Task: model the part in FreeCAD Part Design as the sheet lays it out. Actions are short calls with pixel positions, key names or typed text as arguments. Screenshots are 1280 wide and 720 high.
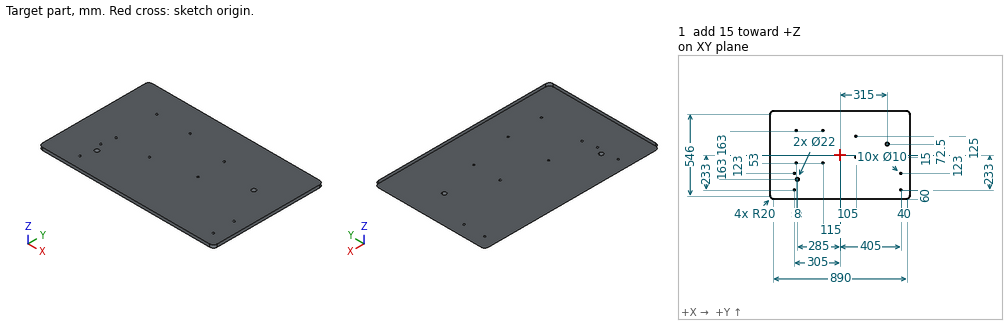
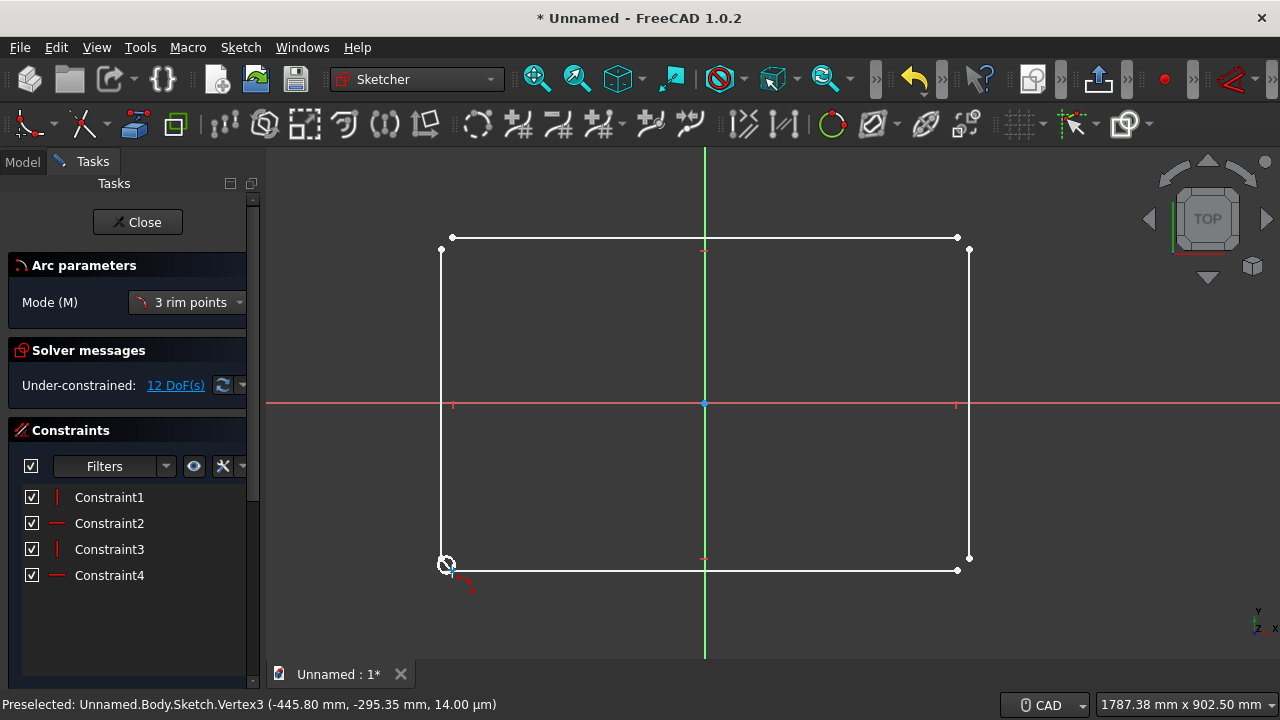
scroll(444, 566, up, 8)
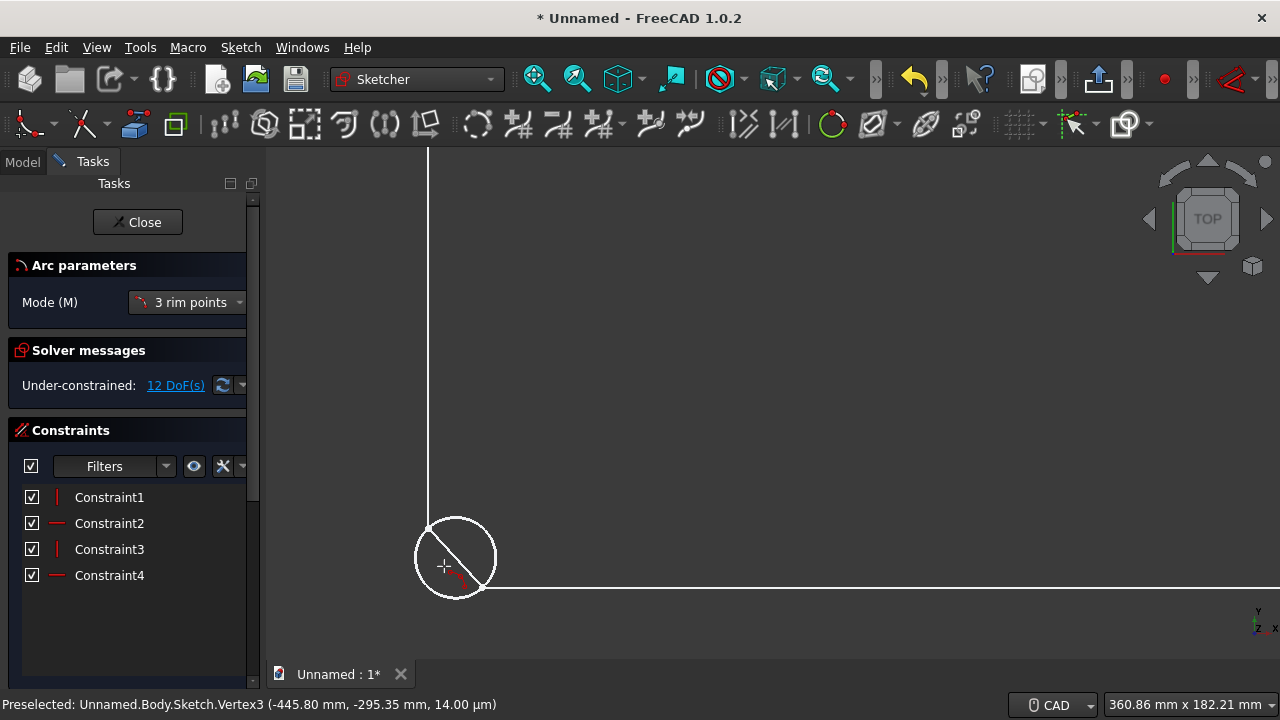
click(445, 564)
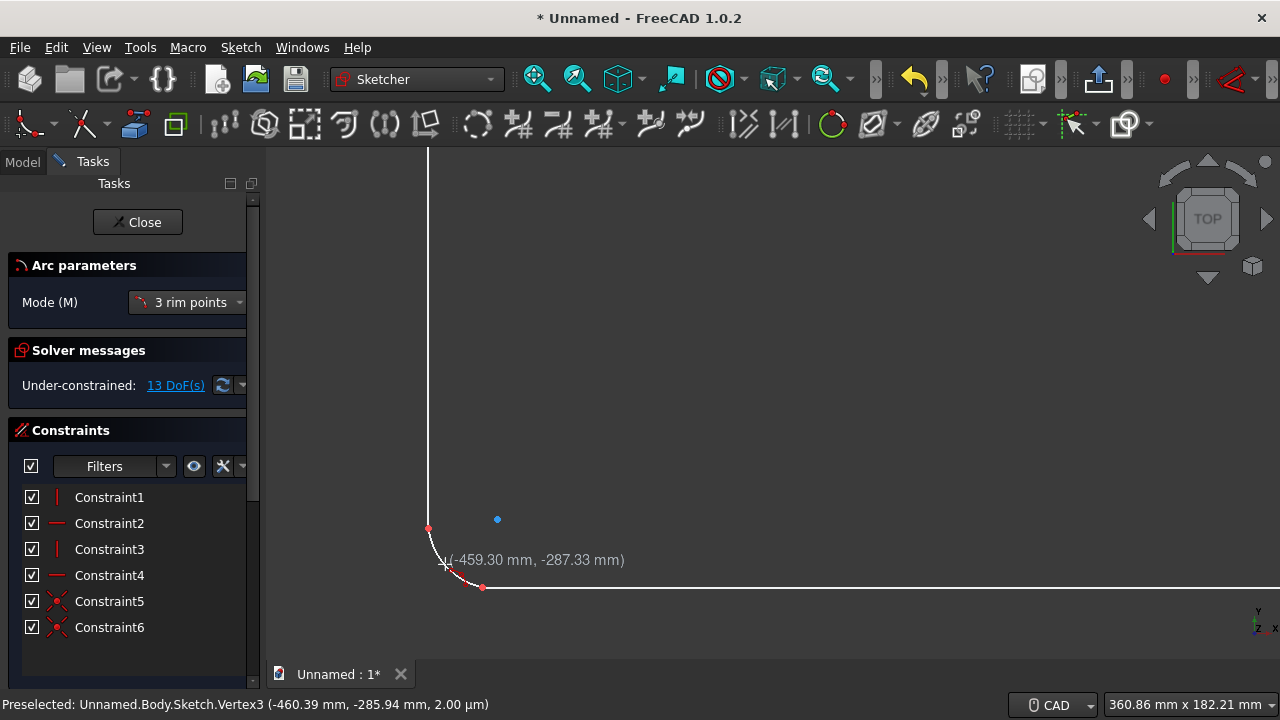
scroll(444, 566, down, 8)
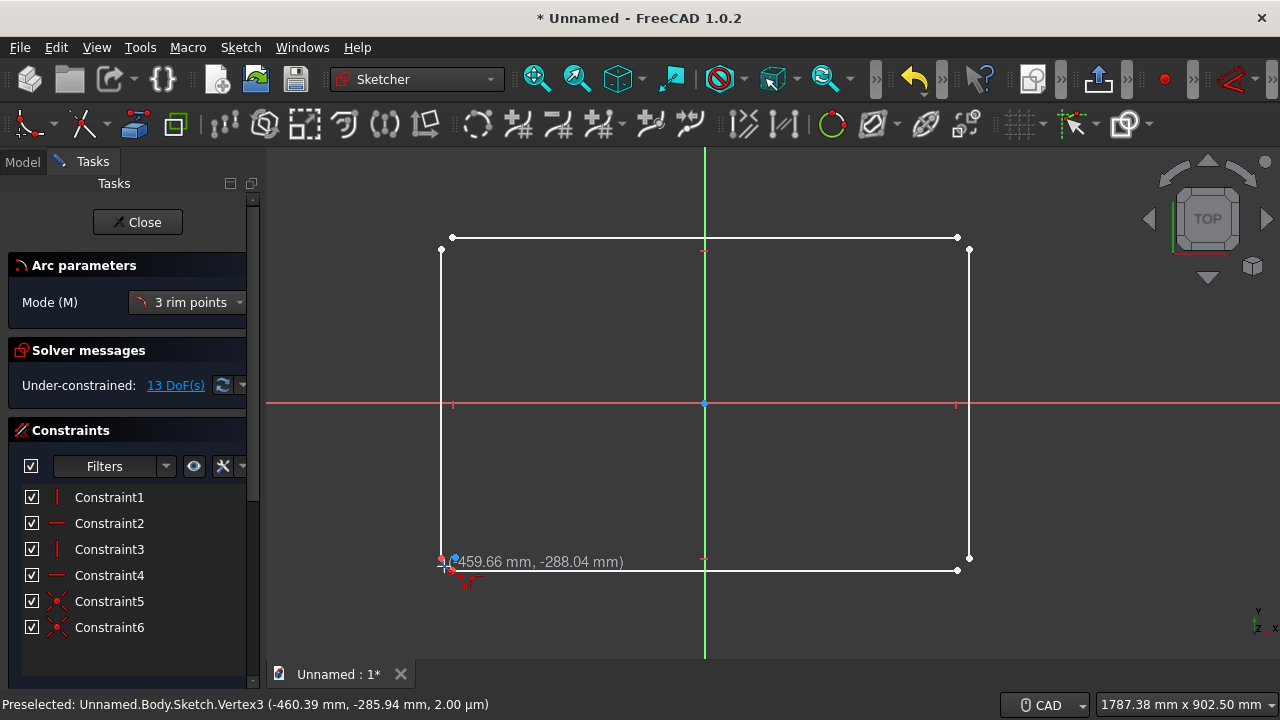
click(957, 571)
click(969, 559)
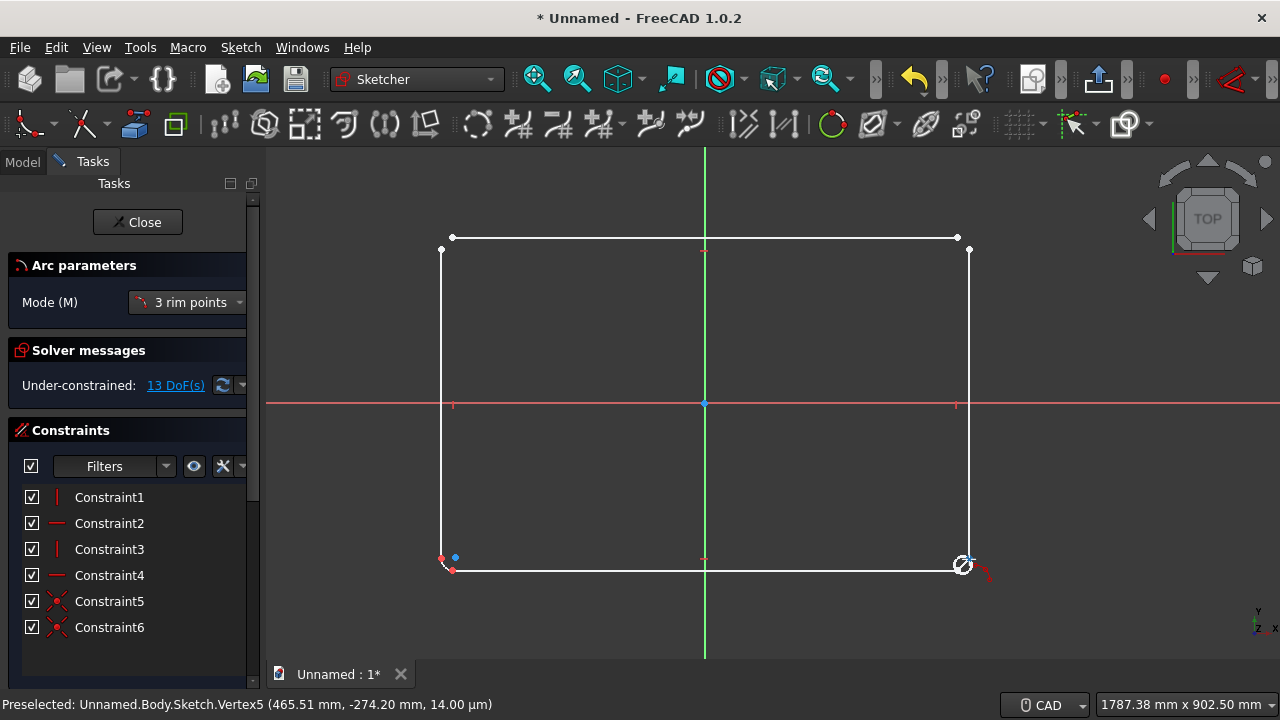
scroll(965, 566, up, 8)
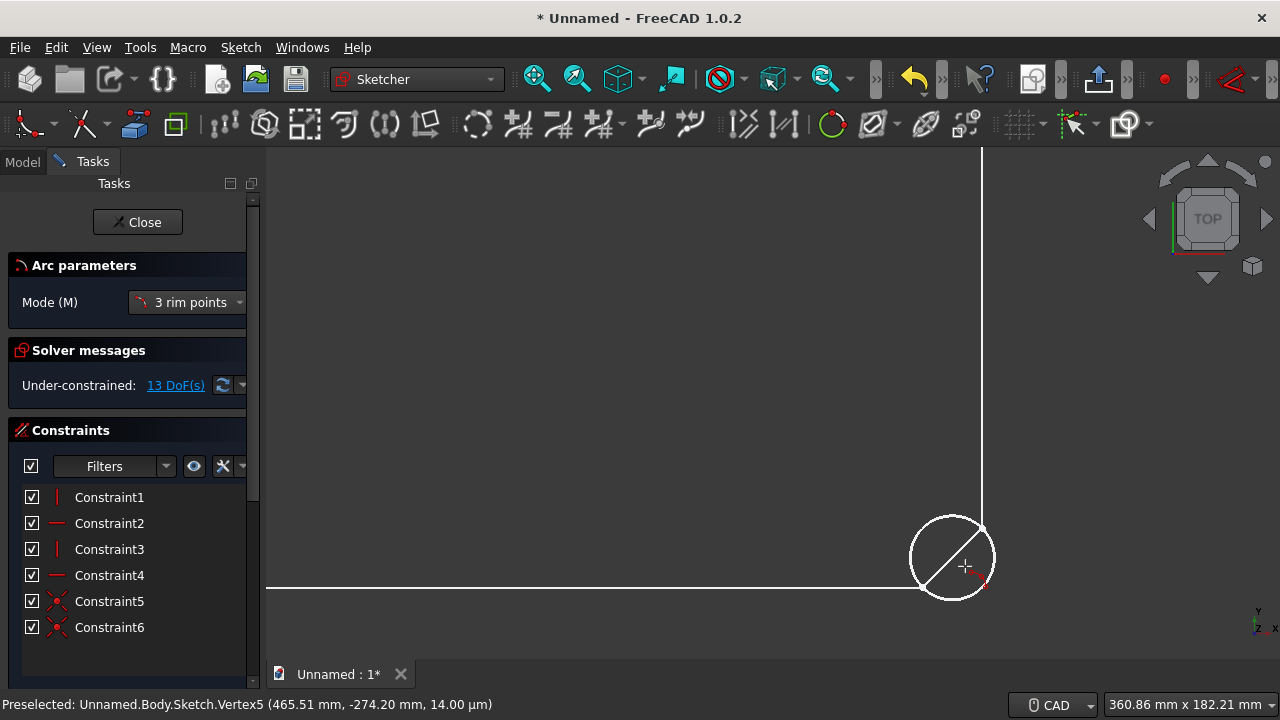
click(964, 564)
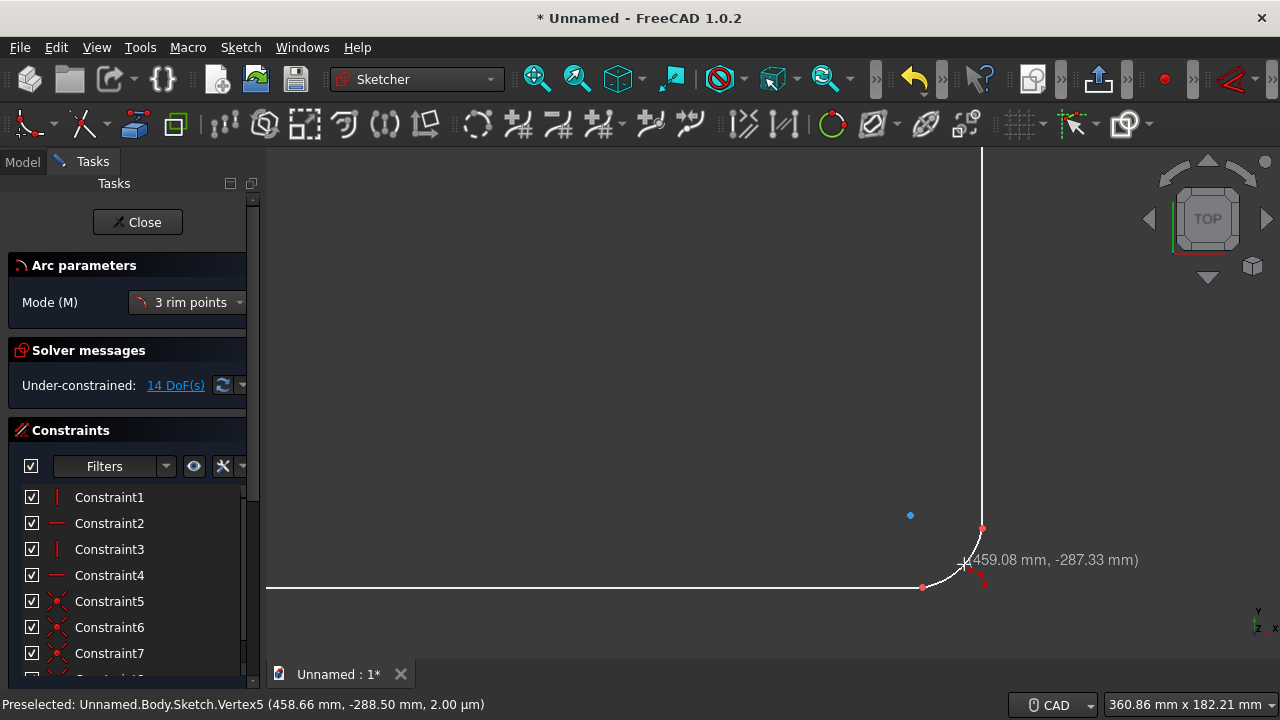
scroll(965, 566, down, 8)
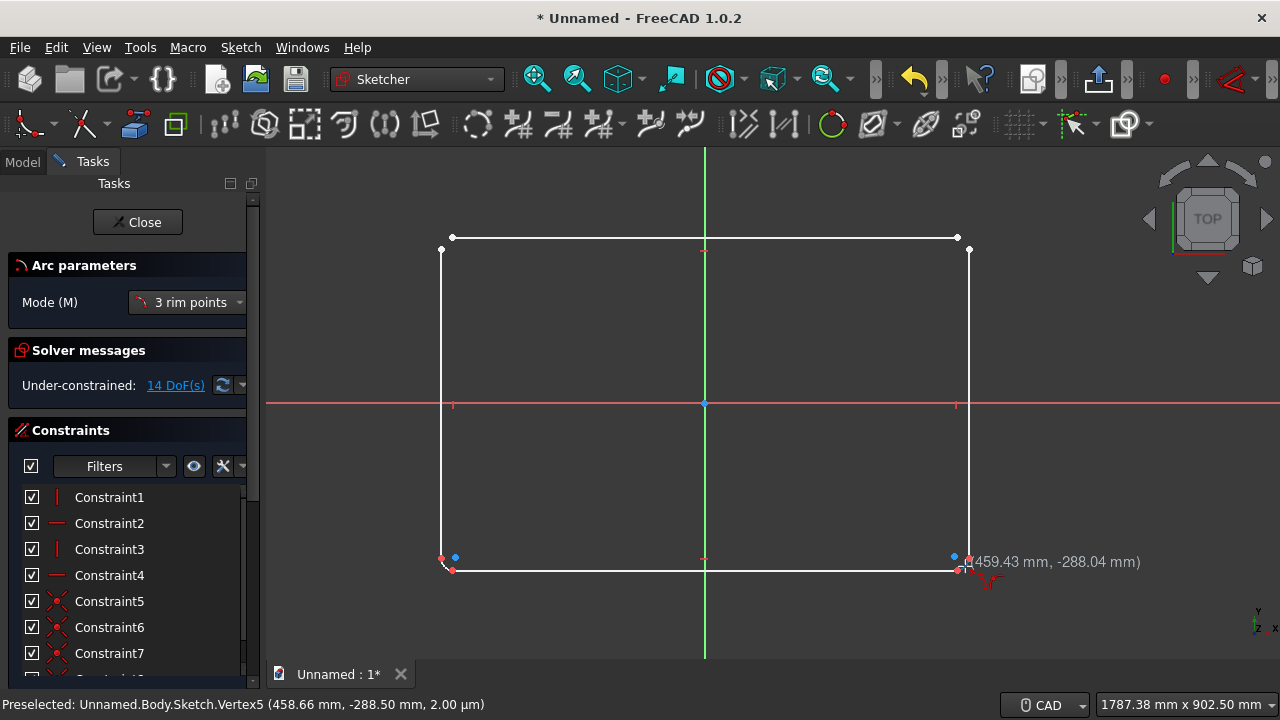
click(969, 250)
click(957, 238)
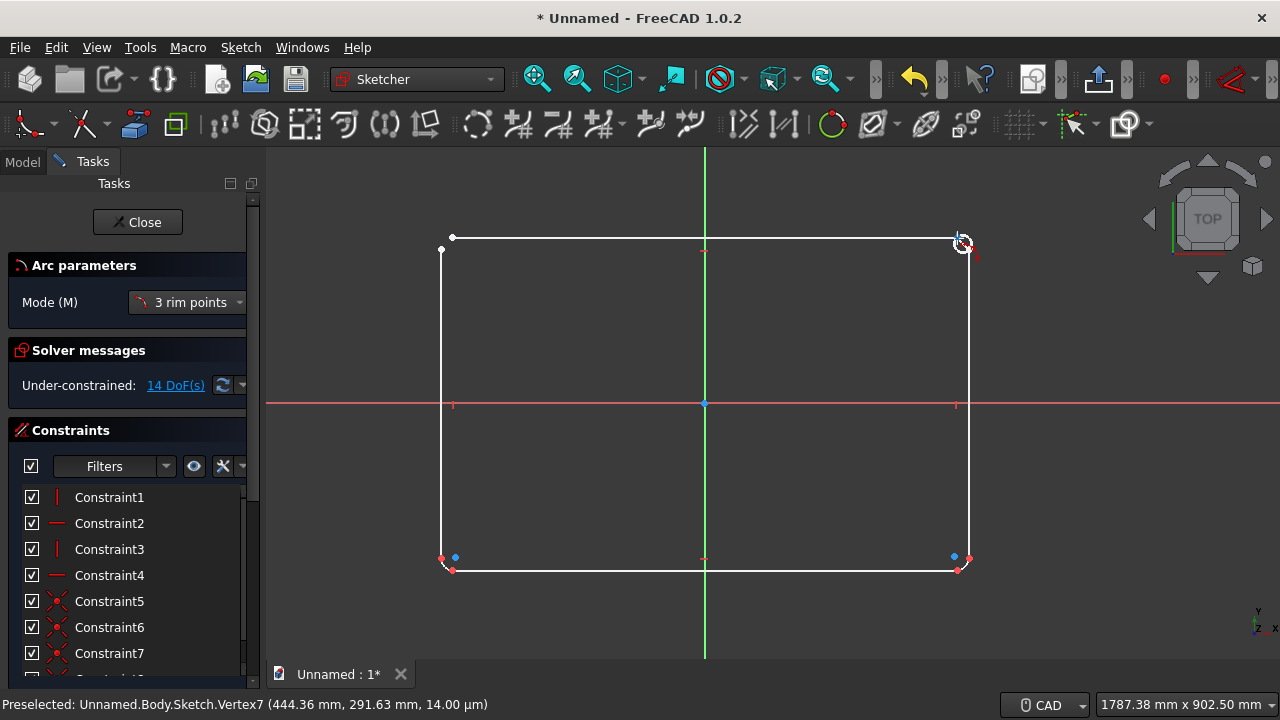
scroll(965, 241, up, 8)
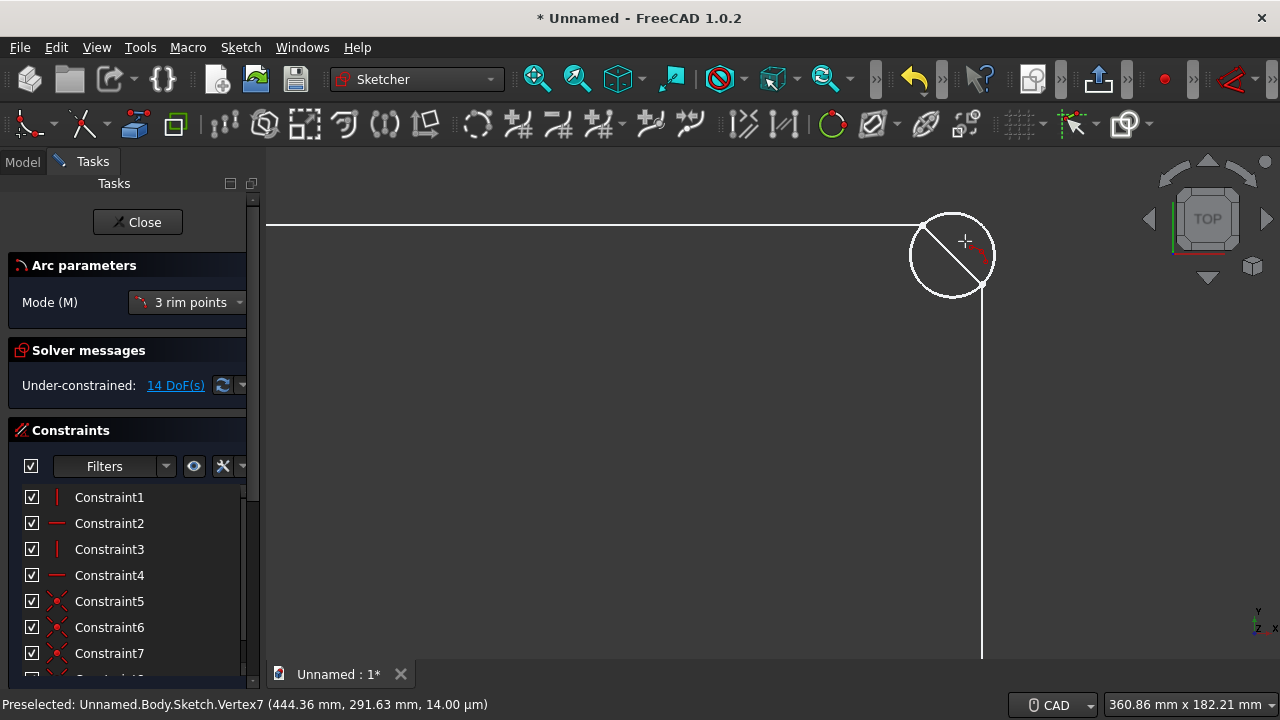
click(964, 238)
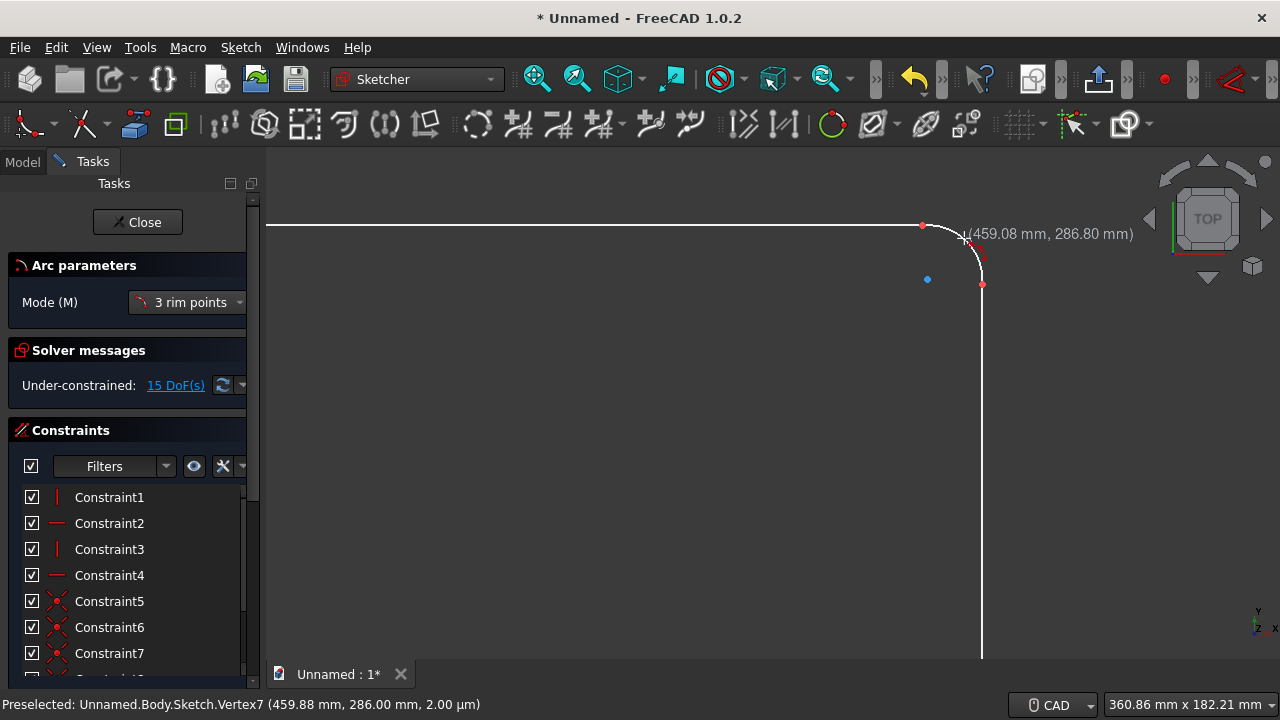
scroll(965, 241, down, 8)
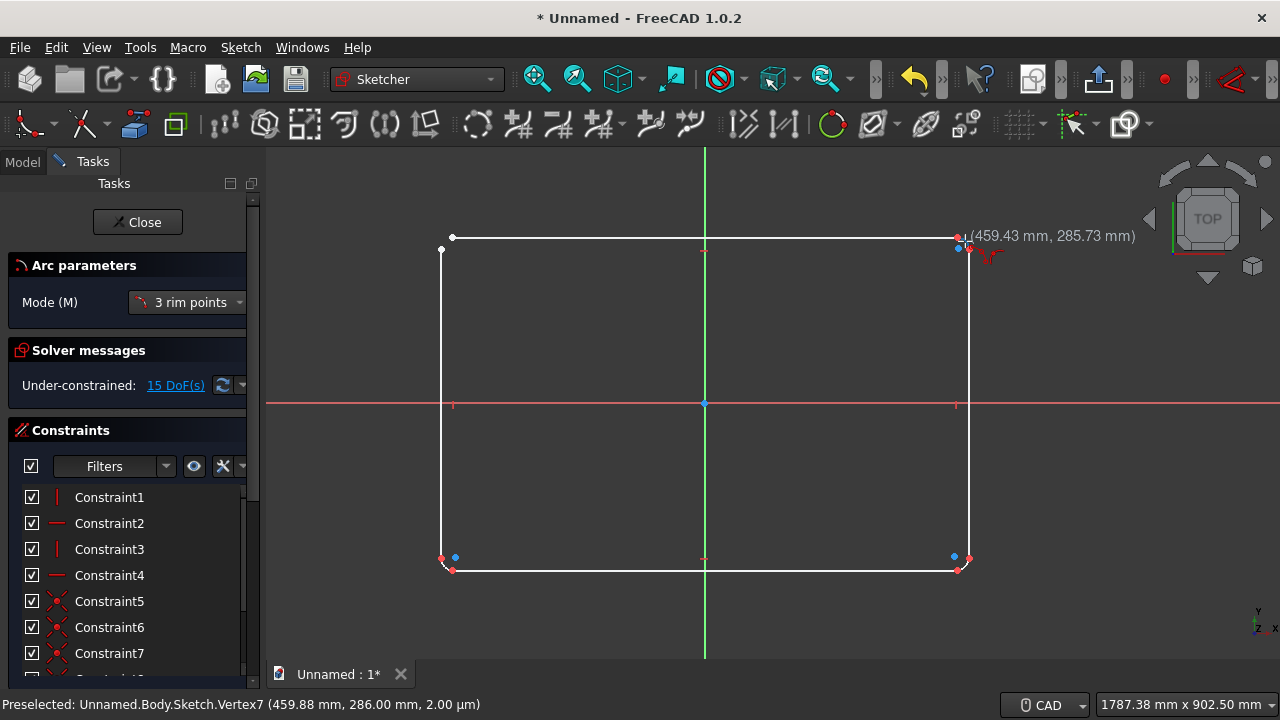
click(452, 238)
click(441, 250)